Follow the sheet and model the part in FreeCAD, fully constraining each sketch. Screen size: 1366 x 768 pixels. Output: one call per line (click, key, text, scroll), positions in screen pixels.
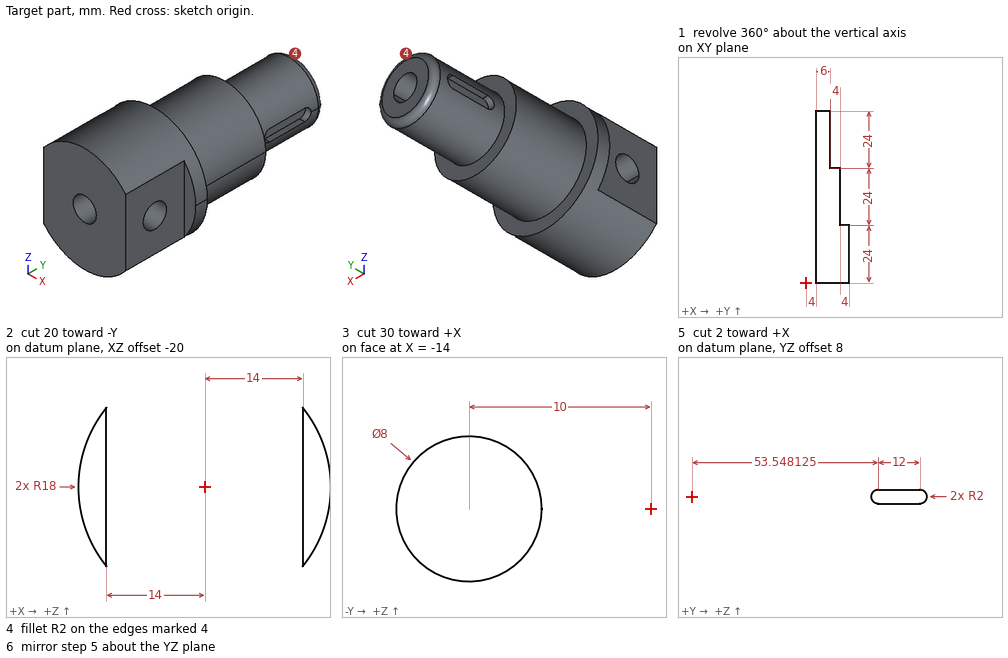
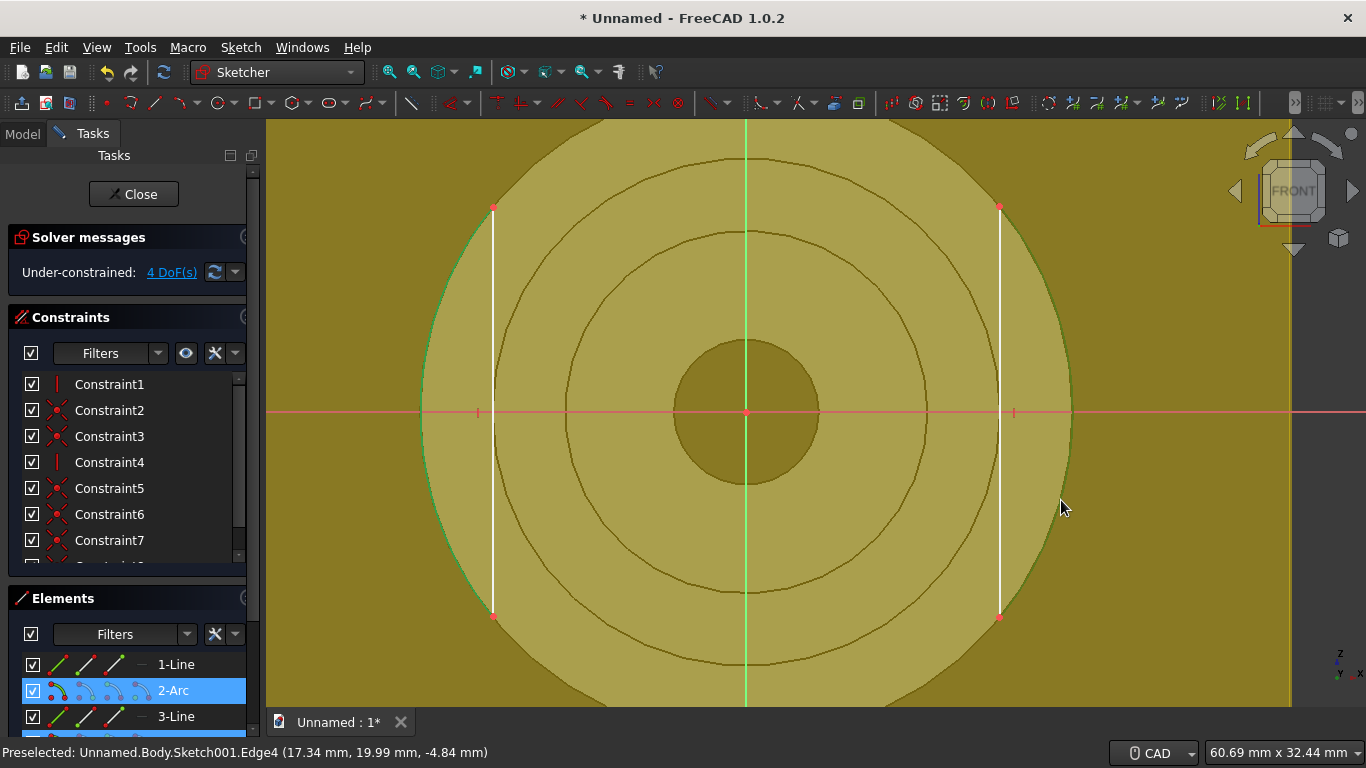
click(630, 104)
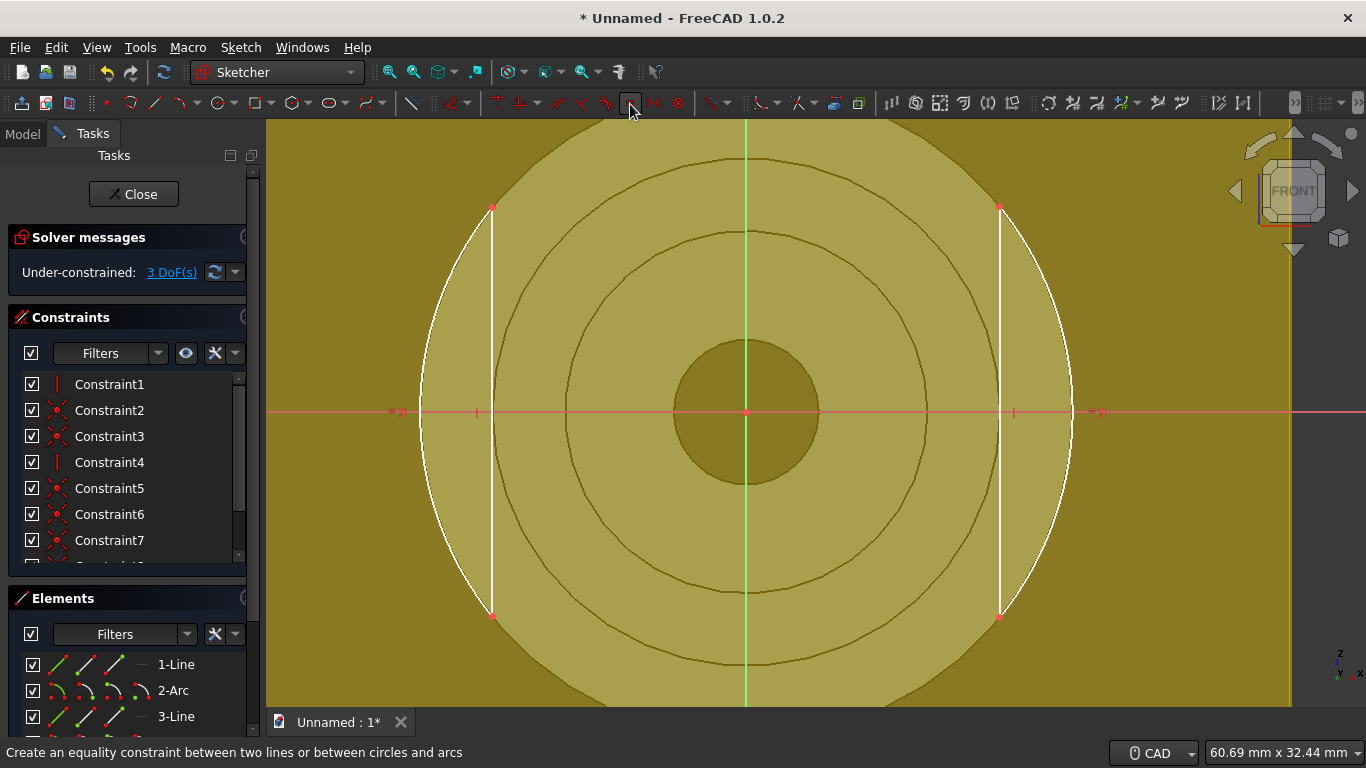
click(450, 104)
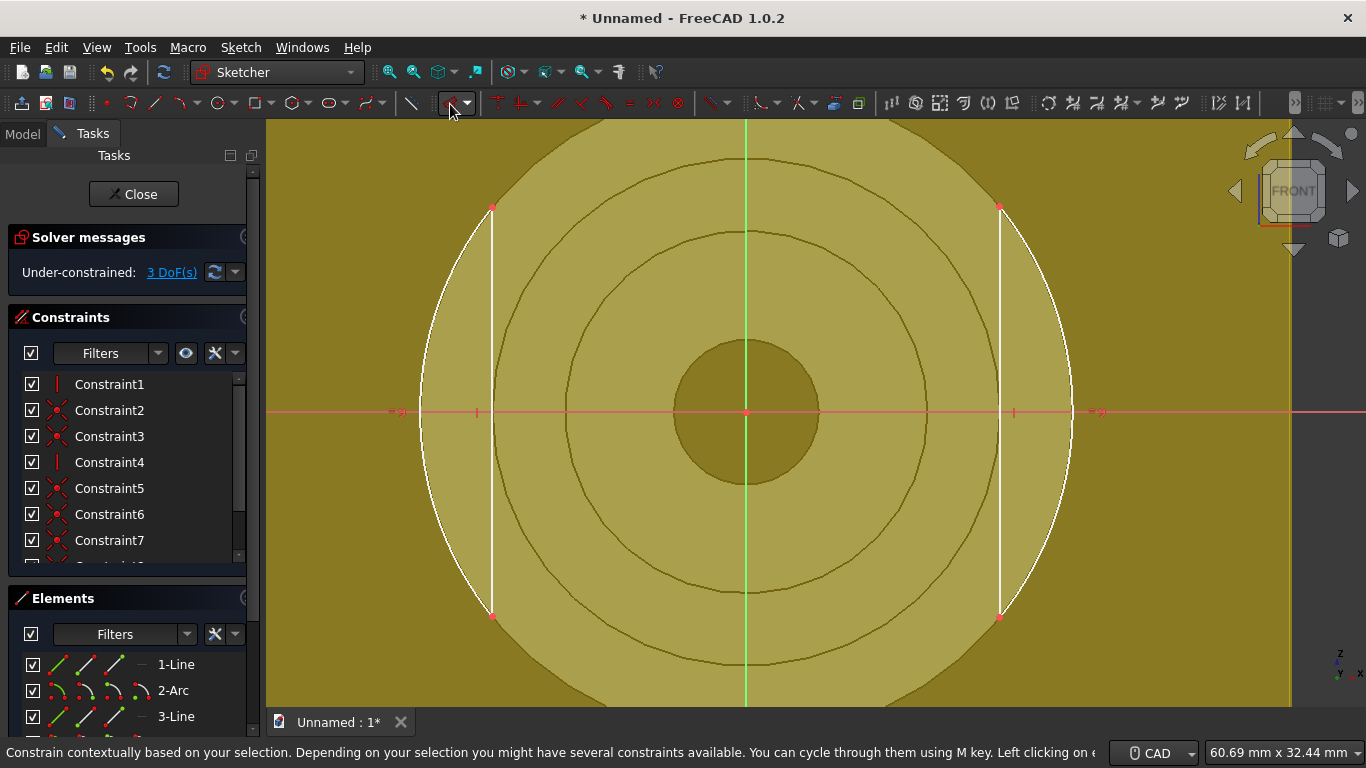
click(432, 325)
click(401, 316)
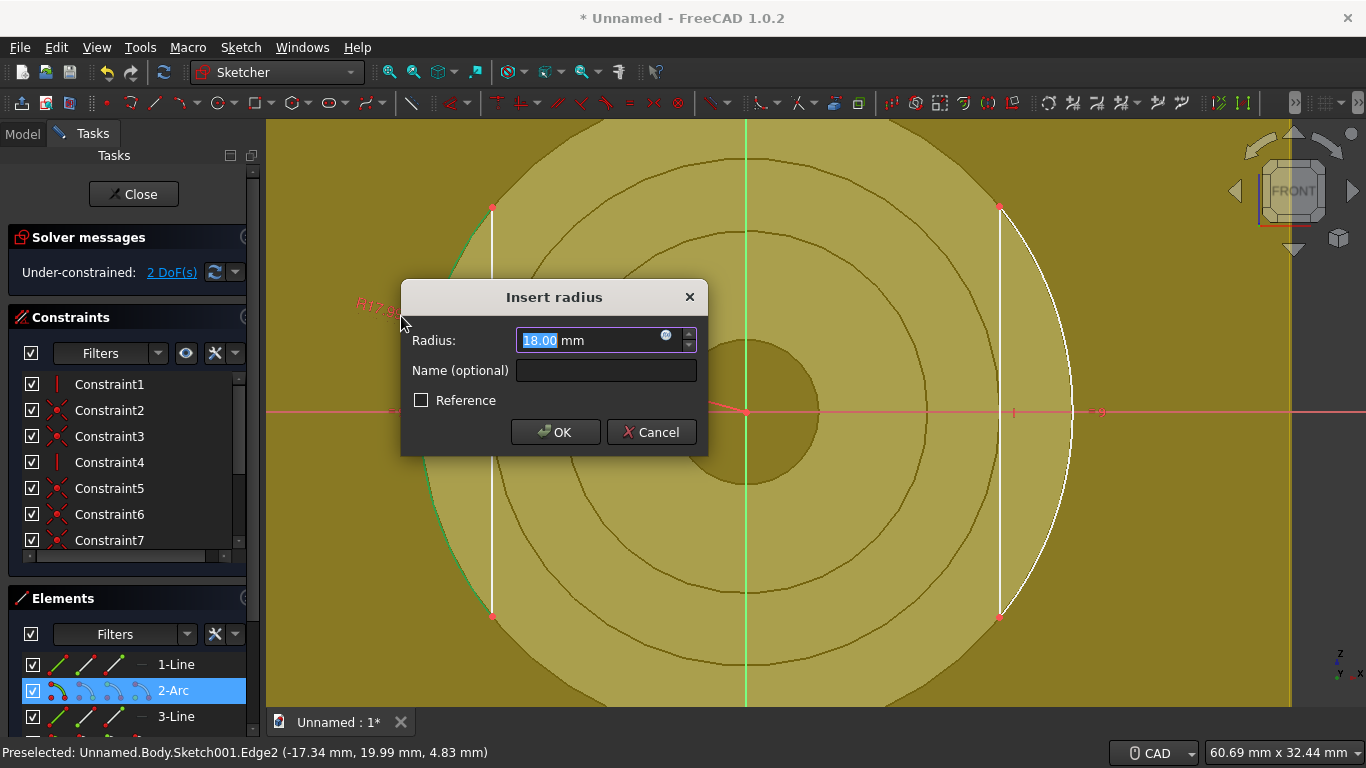
text(18)
key(Return)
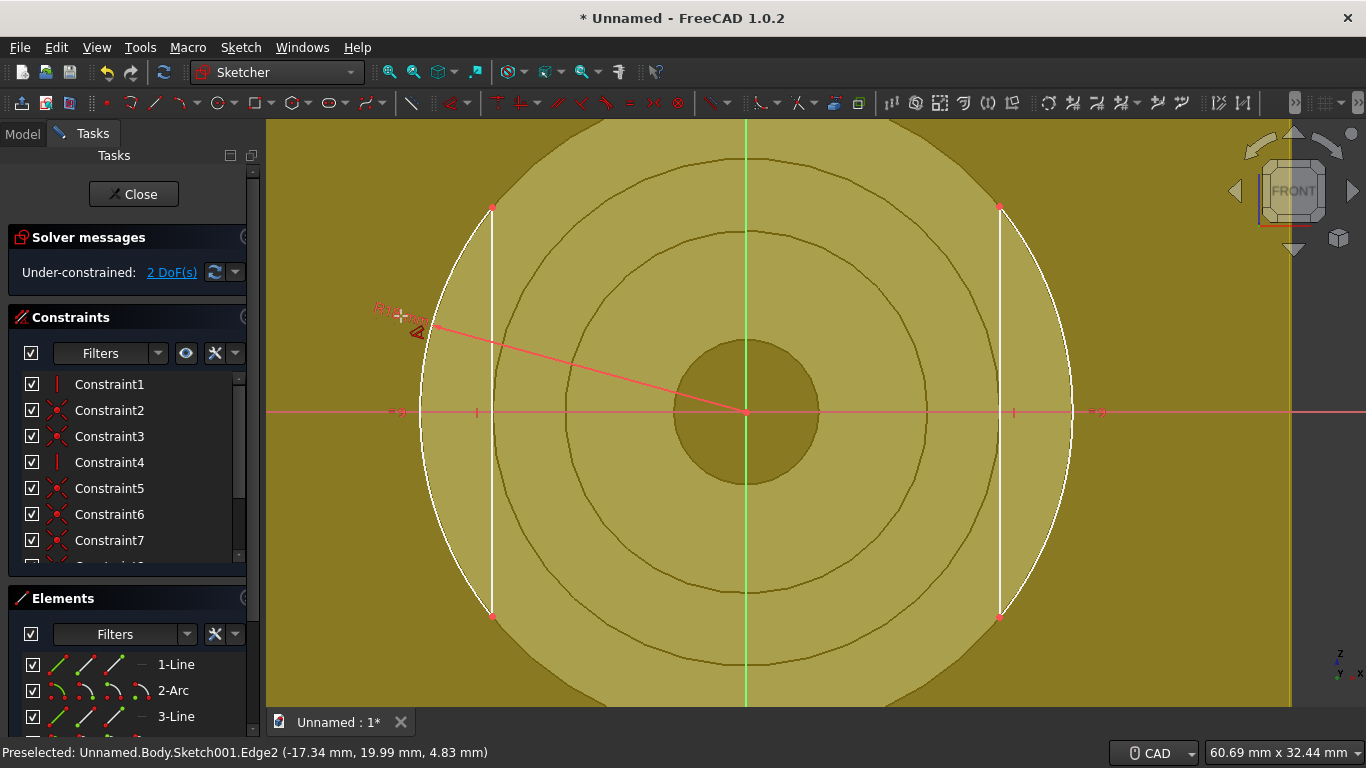
click(492, 617)
click(619, 651)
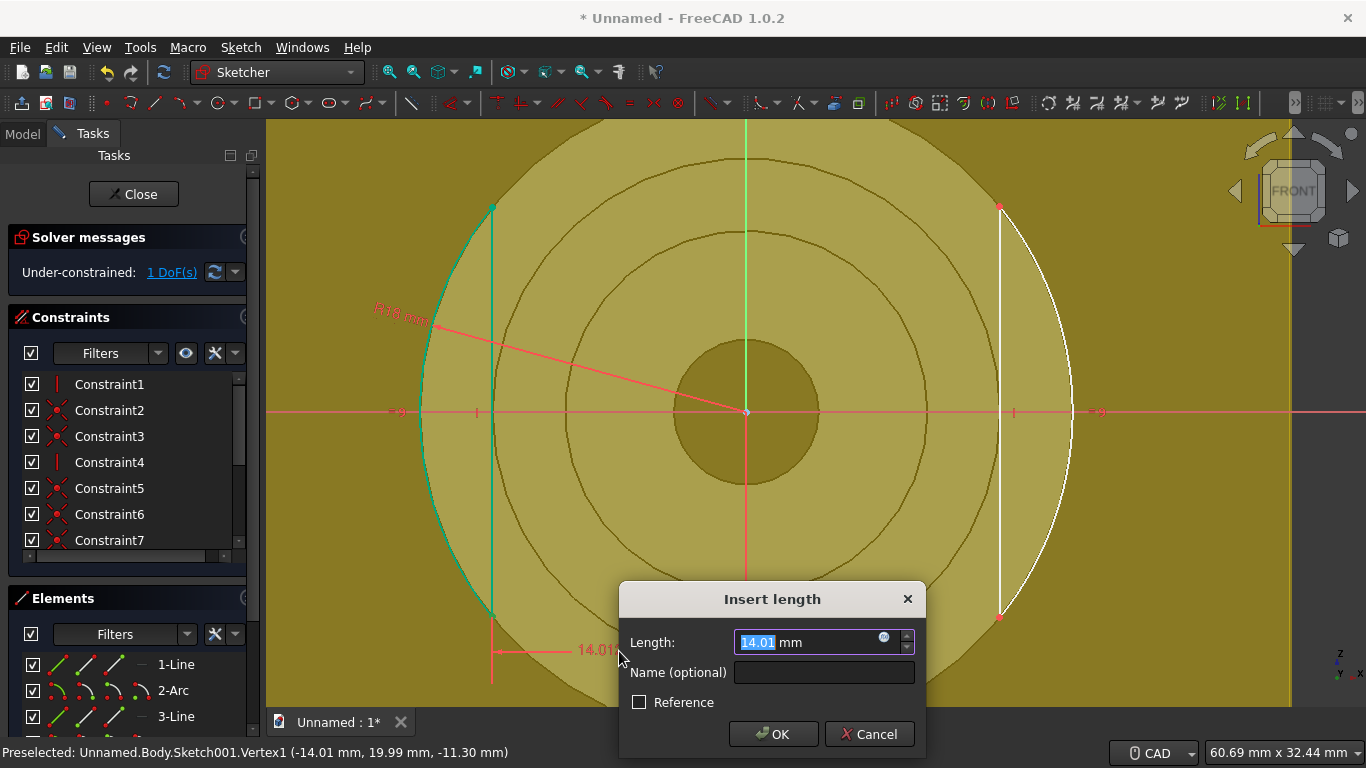
text(14)
key(Return)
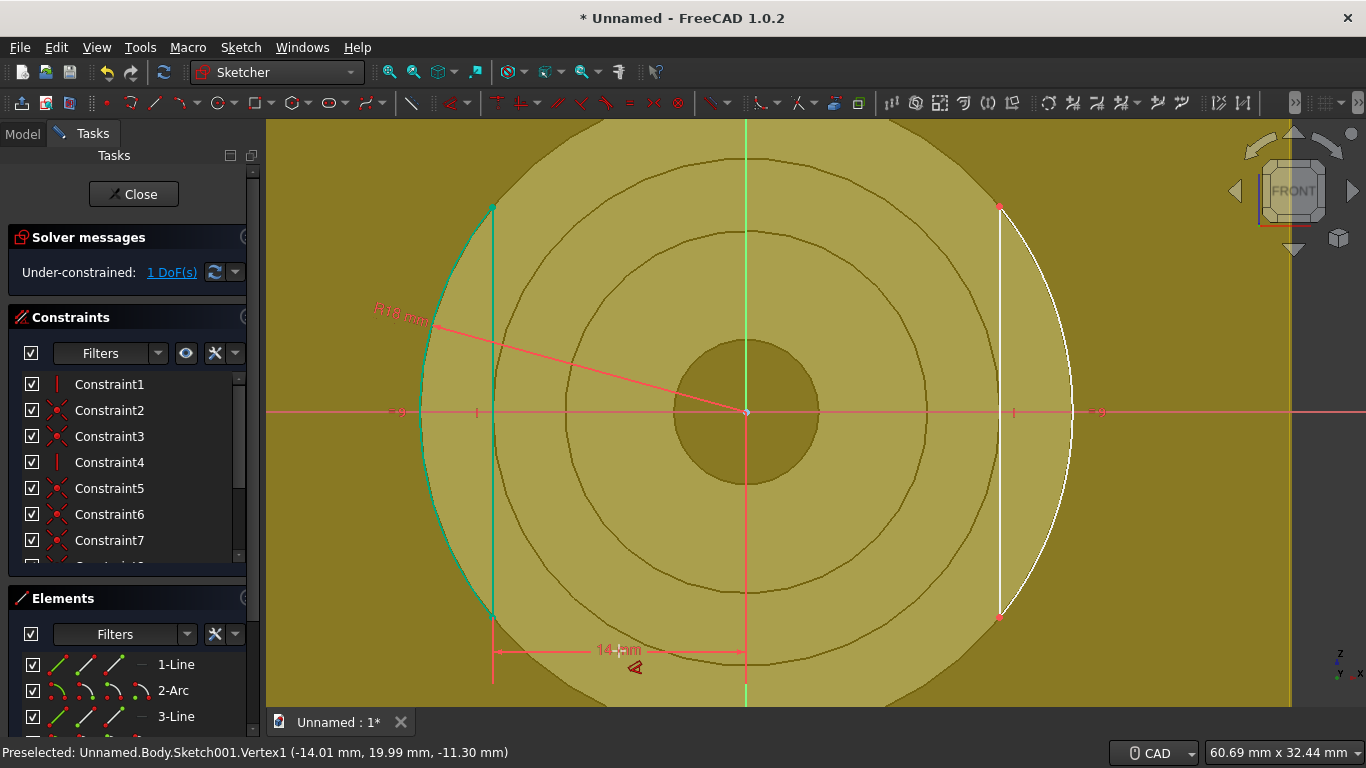
click(1000, 207)
click(873, 173)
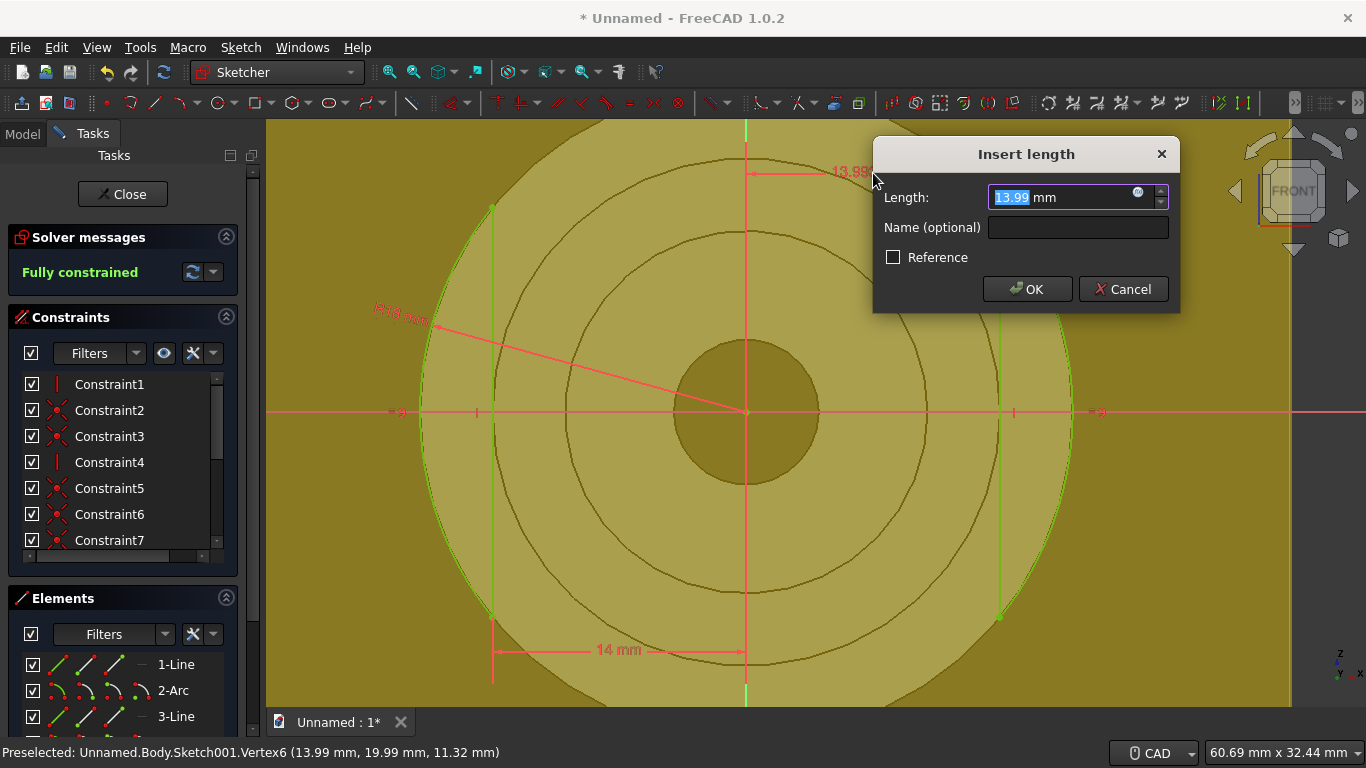
text(14)
key(Return)
key(Escape)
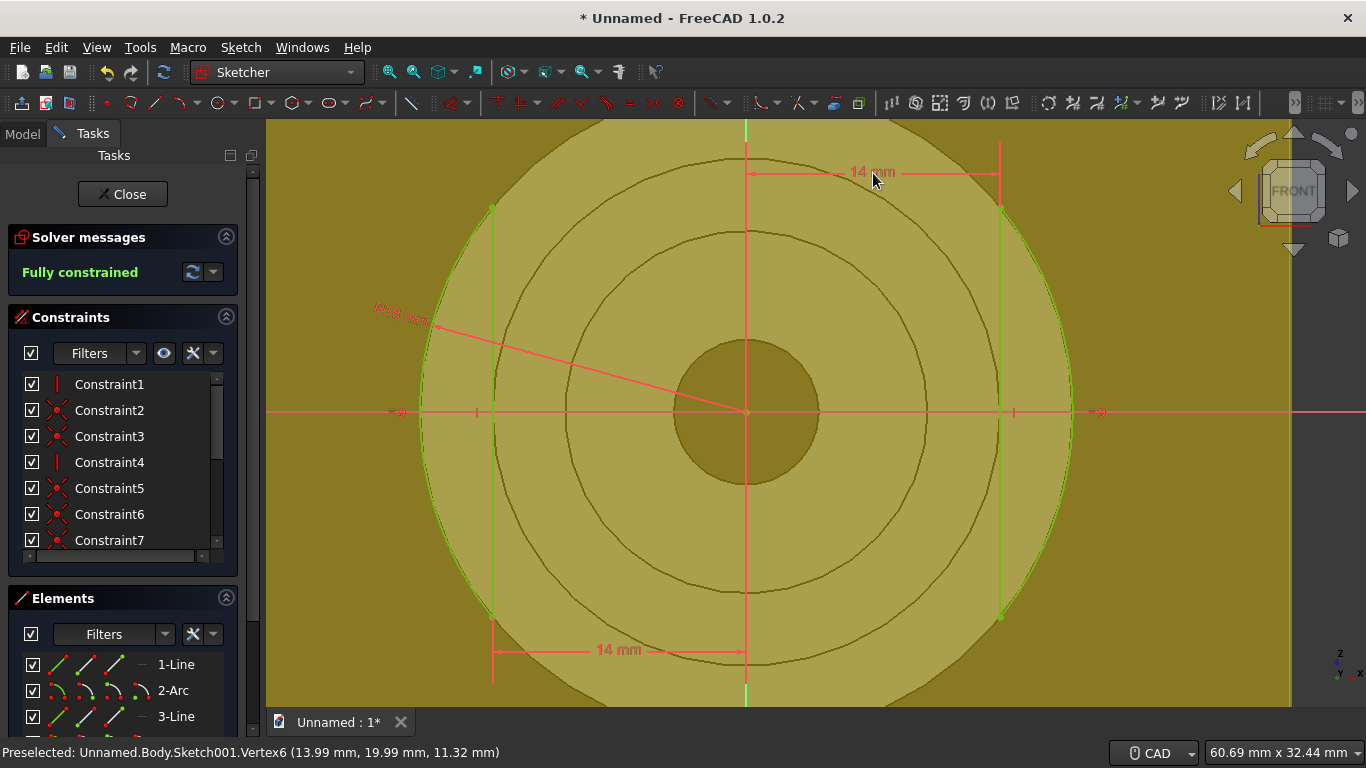
click(123, 194)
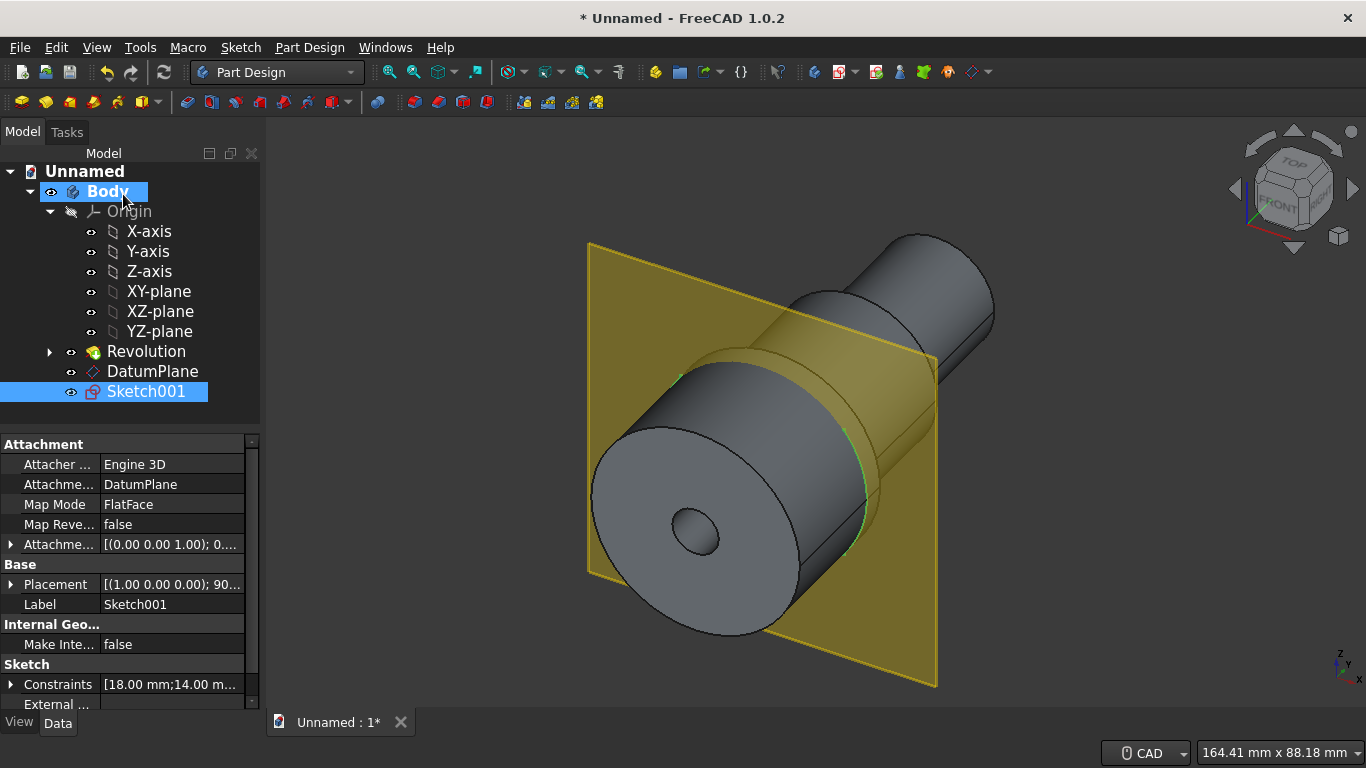
click(188, 102)